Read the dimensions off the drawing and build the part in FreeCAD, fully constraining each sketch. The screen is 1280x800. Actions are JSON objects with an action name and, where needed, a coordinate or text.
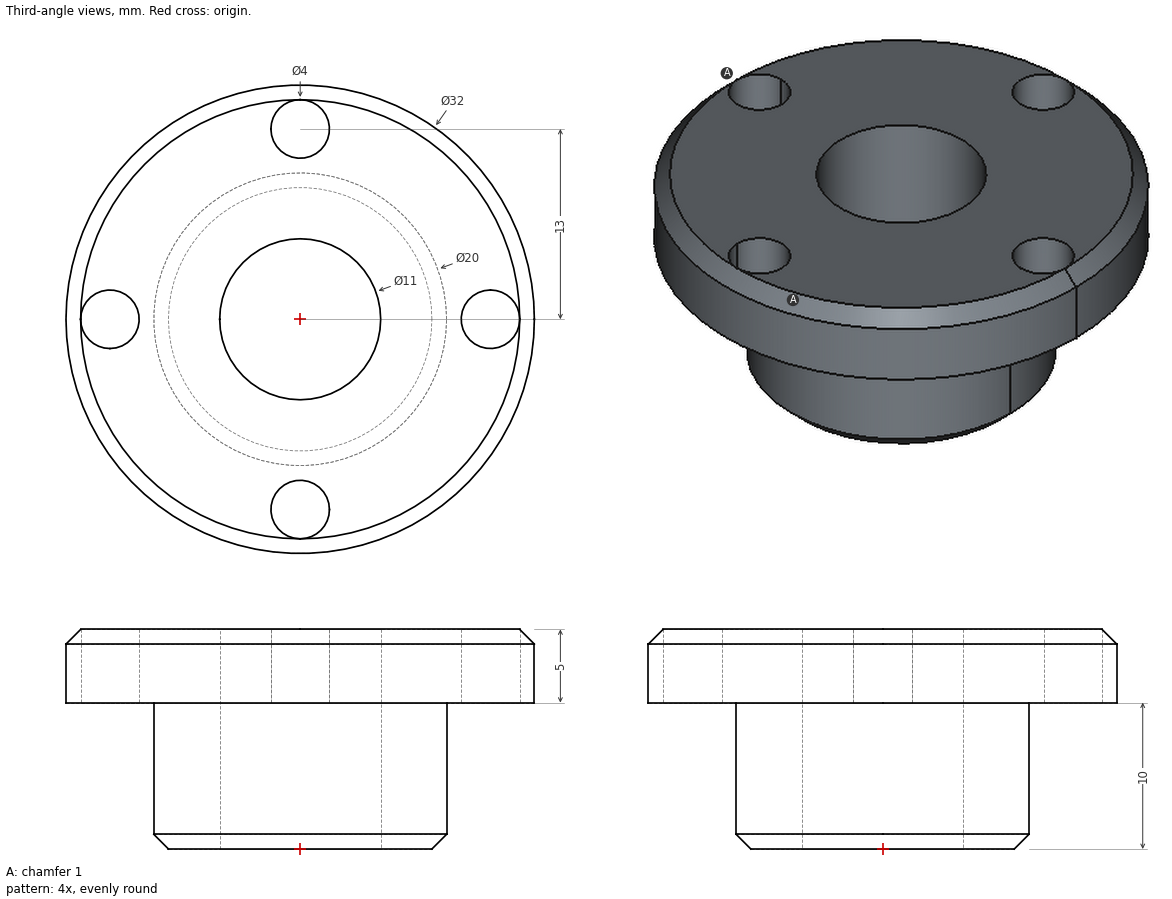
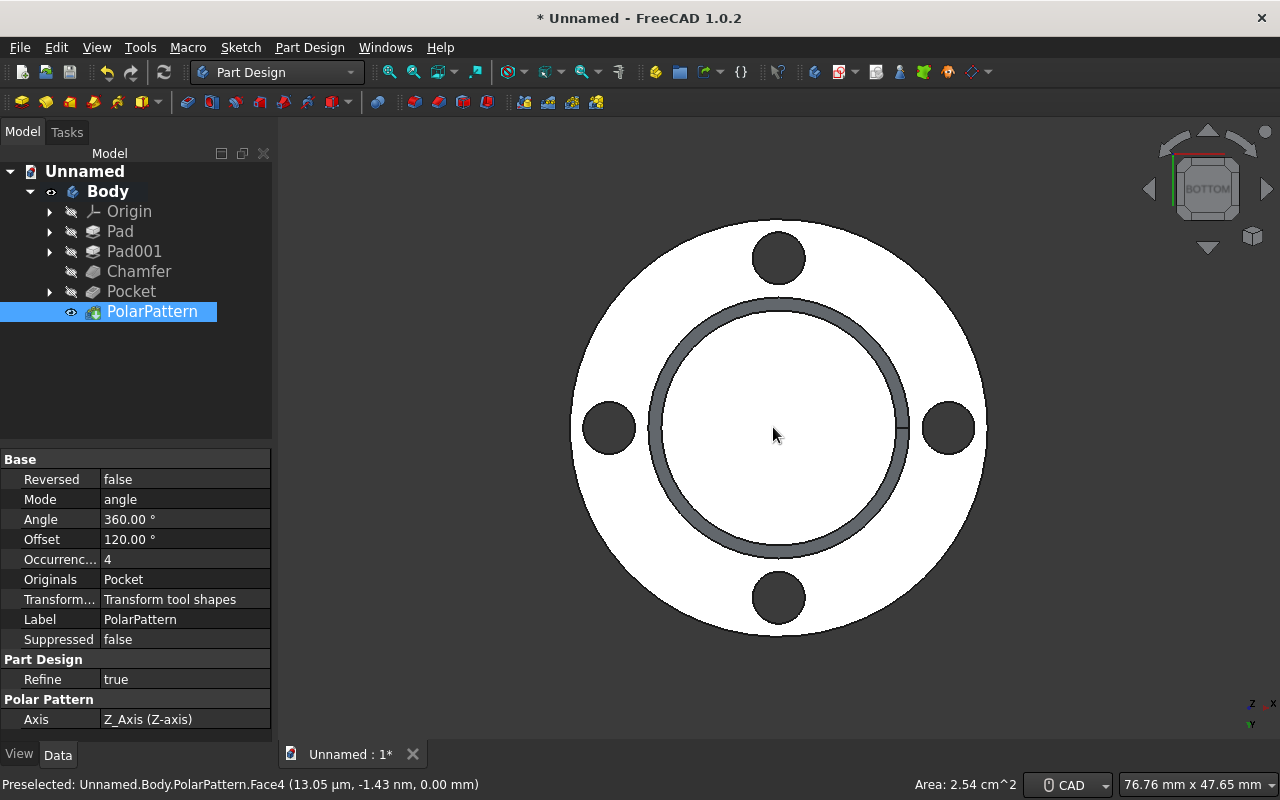
{"action": "left_click", "coordinate": [840, 72]}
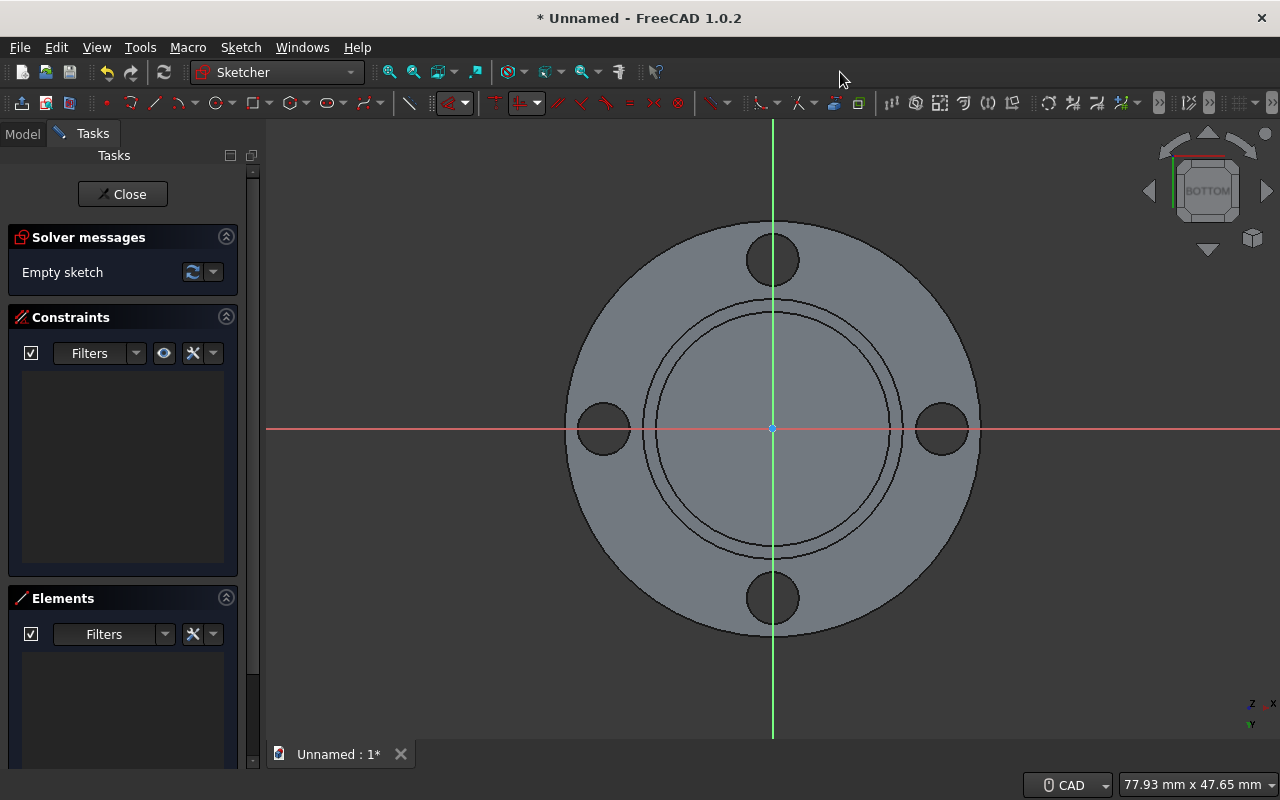
{"action": "scroll", "coordinate": [813, 429], "scroll_direction": "up", "scroll_amount": 5}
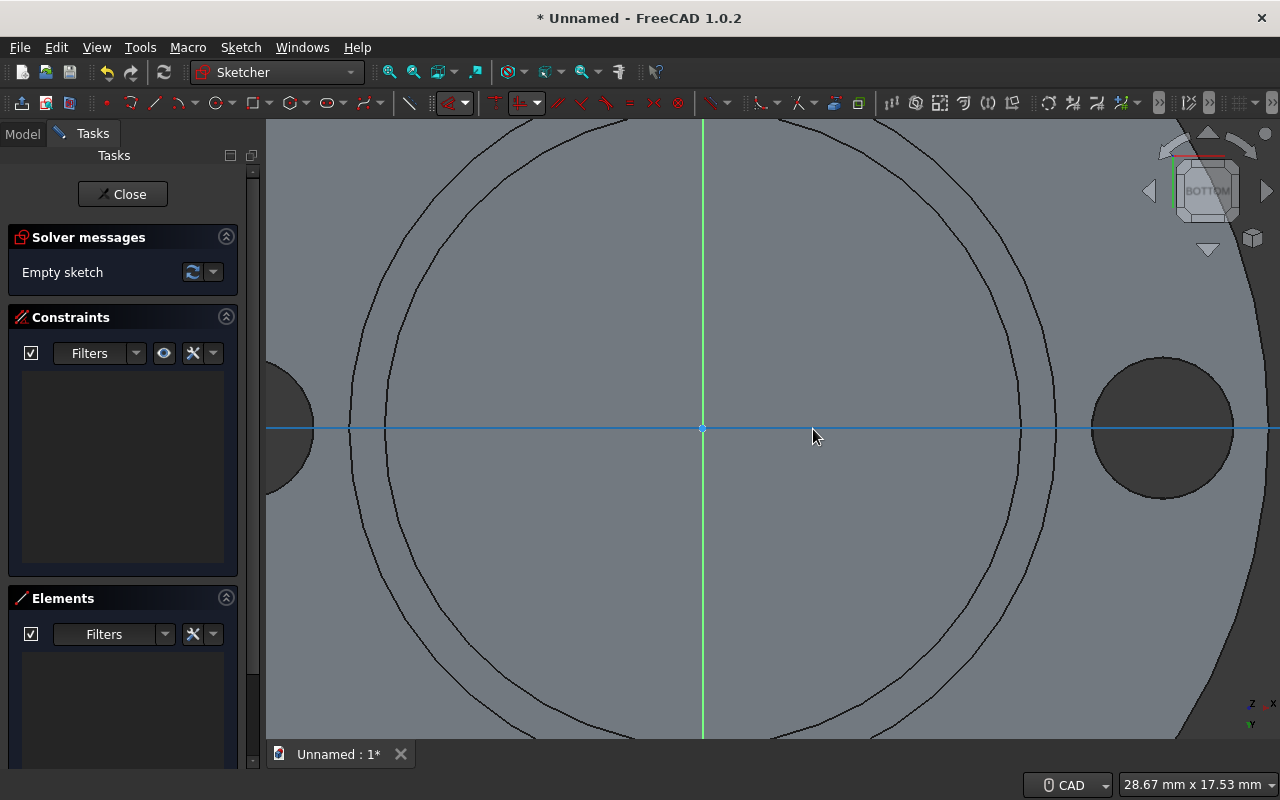
{"action": "left_click", "coordinate": [216, 104]}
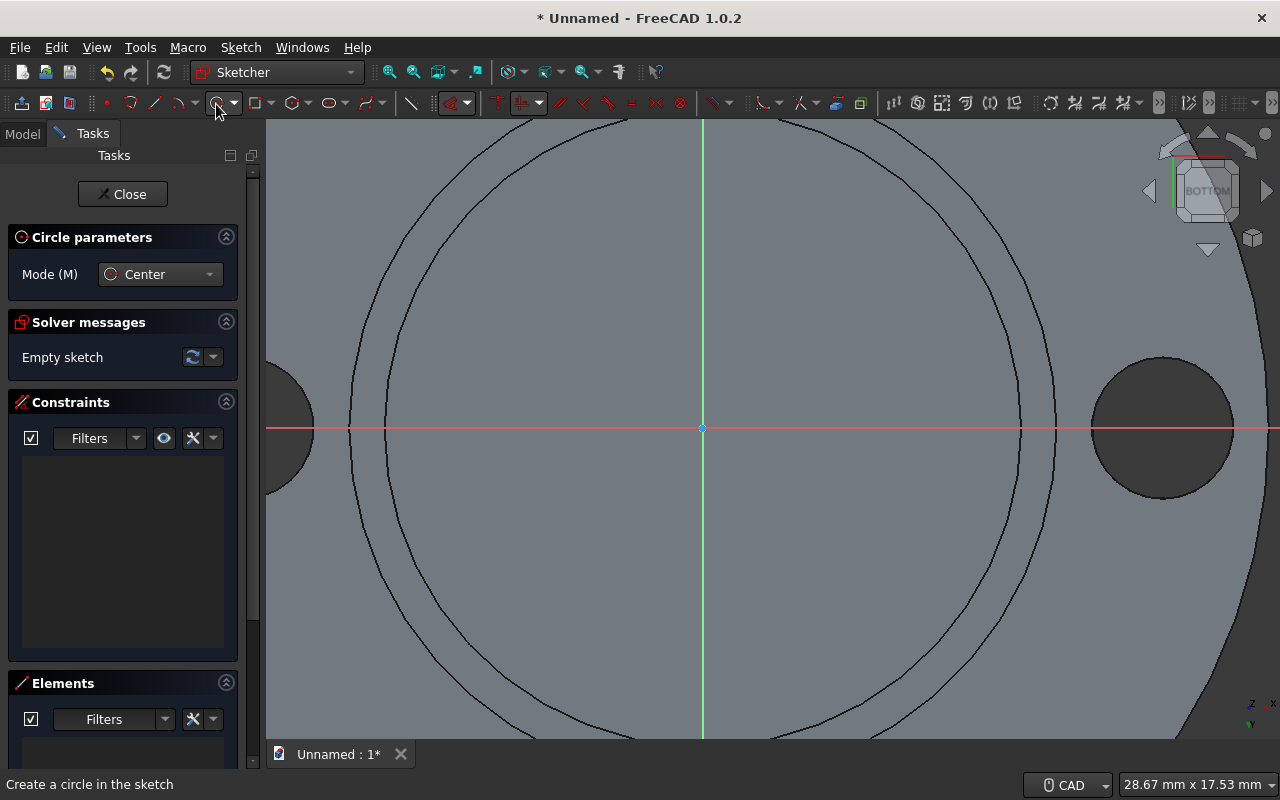
{"action": "left_click", "coordinate": [703, 428]}
{"action": "left_click", "coordinate": [840, 291]}
{"action": "key", "text": "Escape"}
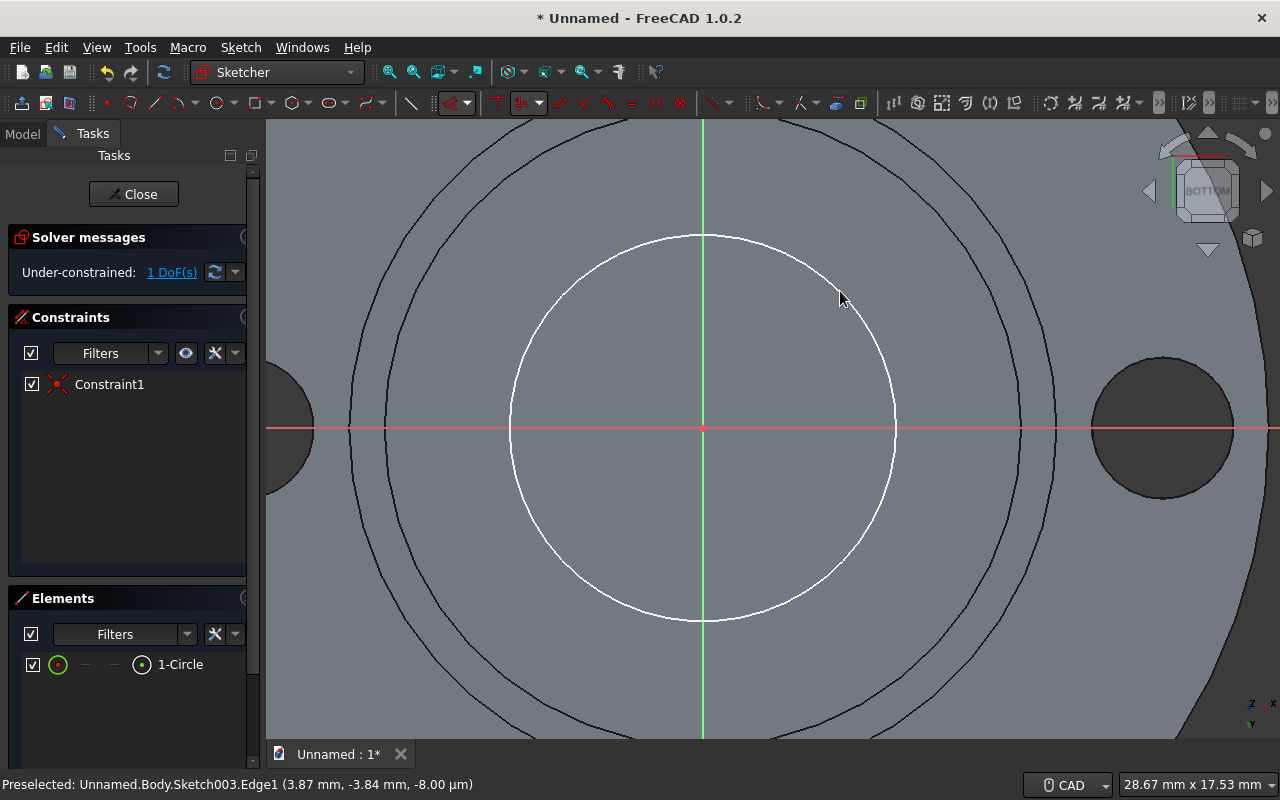
{"action": "left_click", "coordinate": [839, 291]}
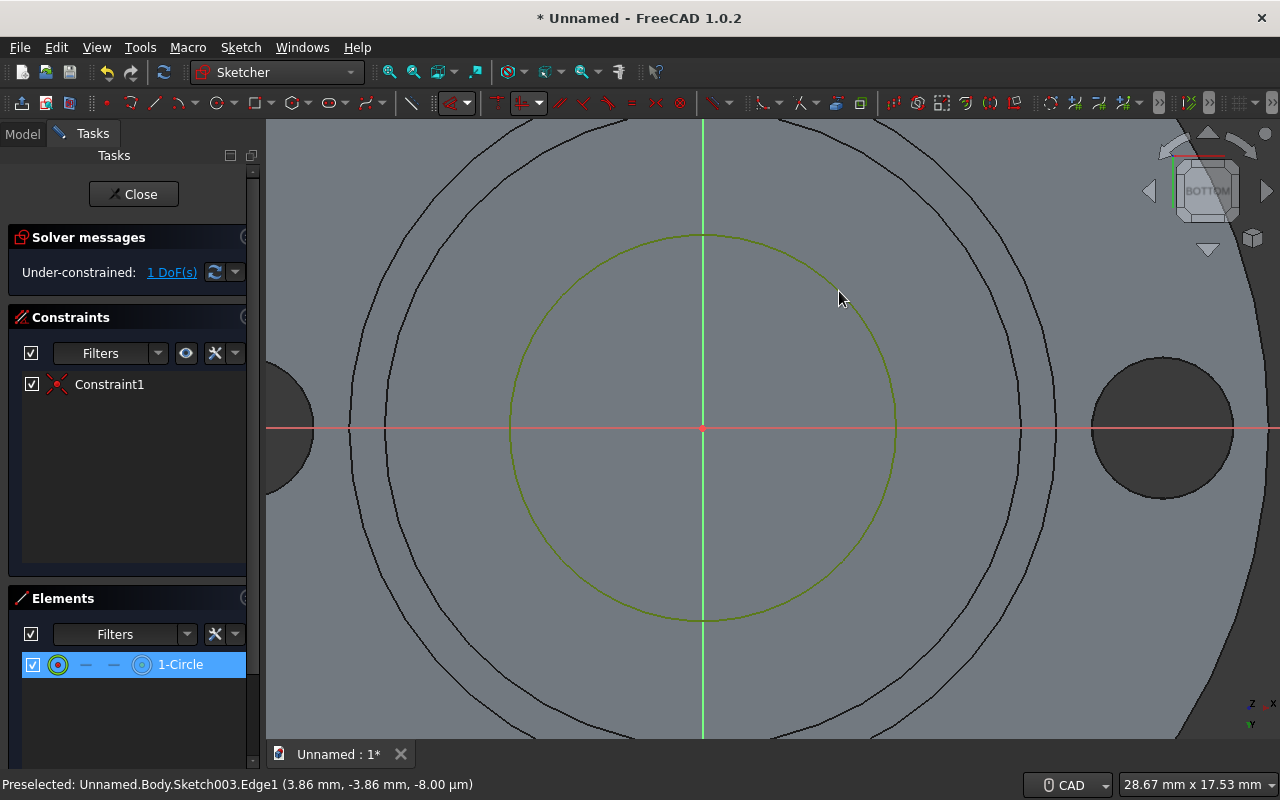
{"action": "left_click", "coordinate": [470, 104]}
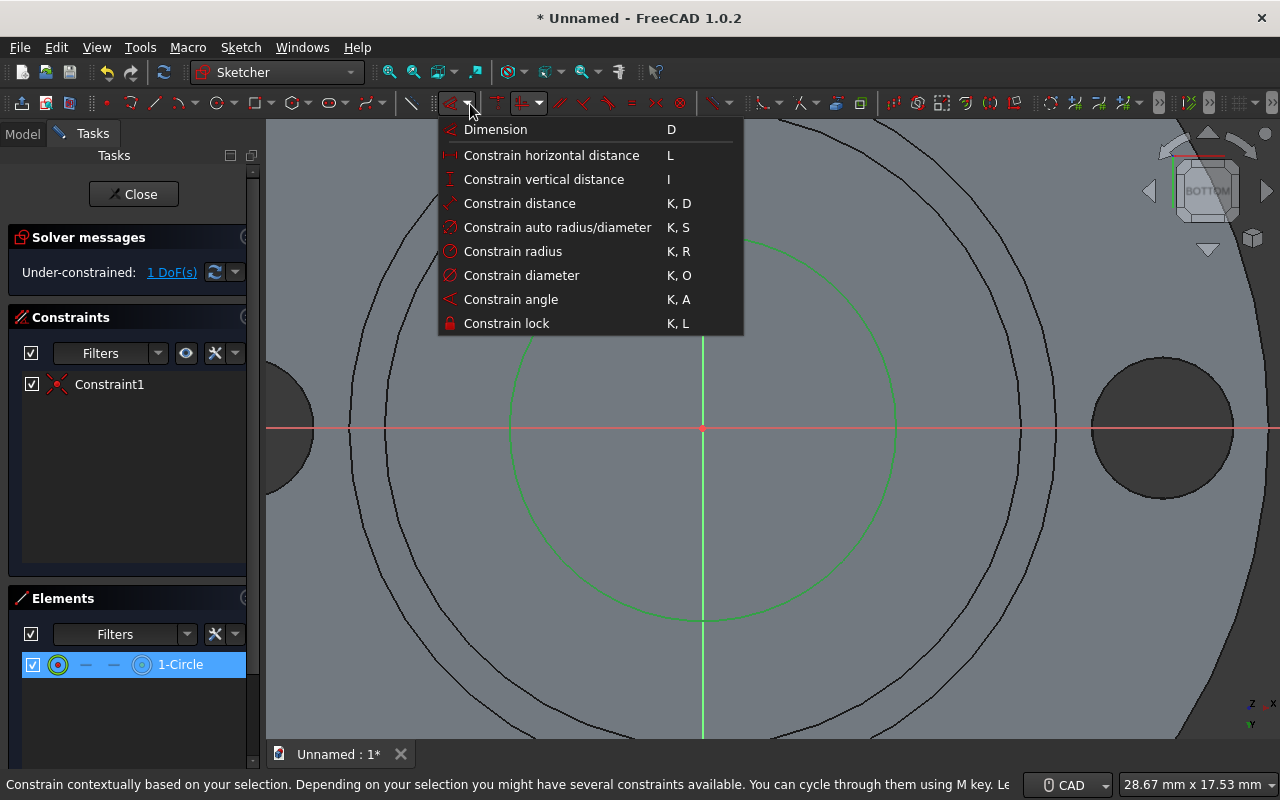
{"action": "left_click", "coordinate": [591, 275]}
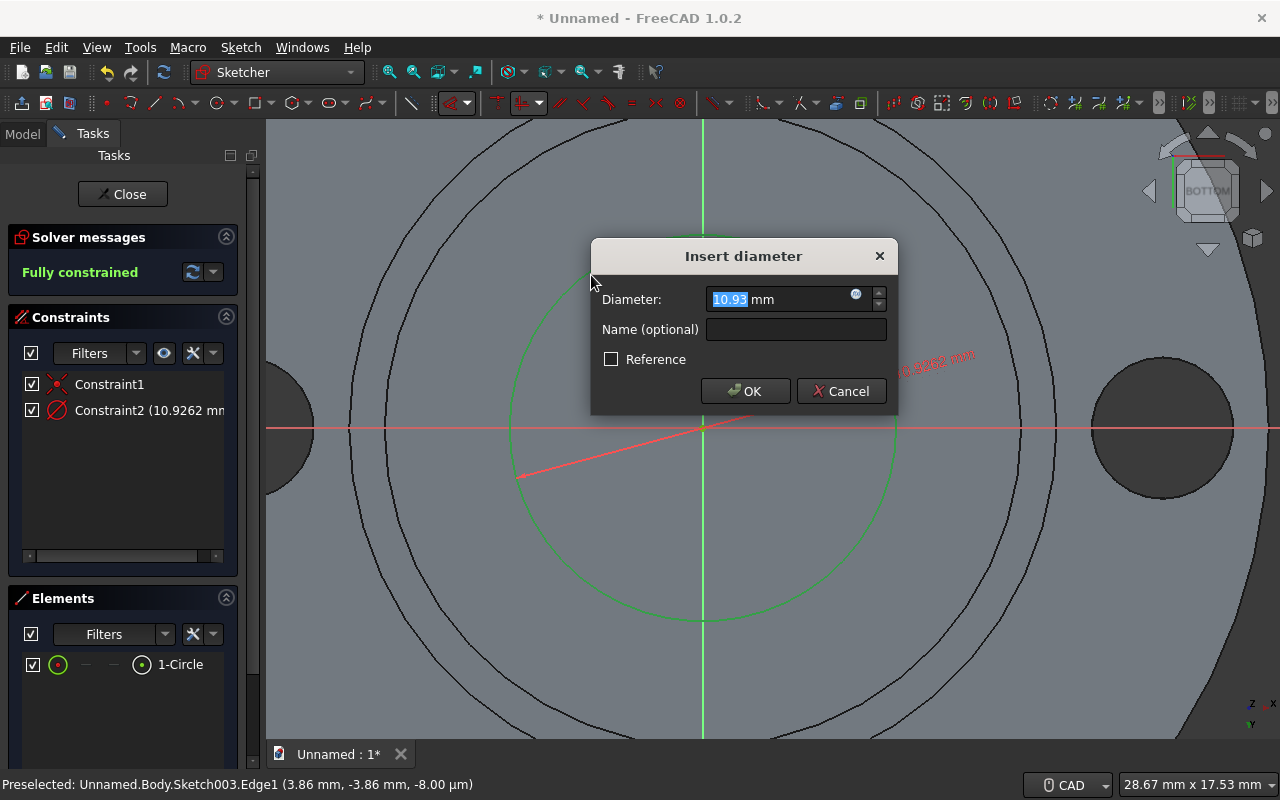
{"action": "type", "text": "11"}
{"action": "key", "text": "Return"}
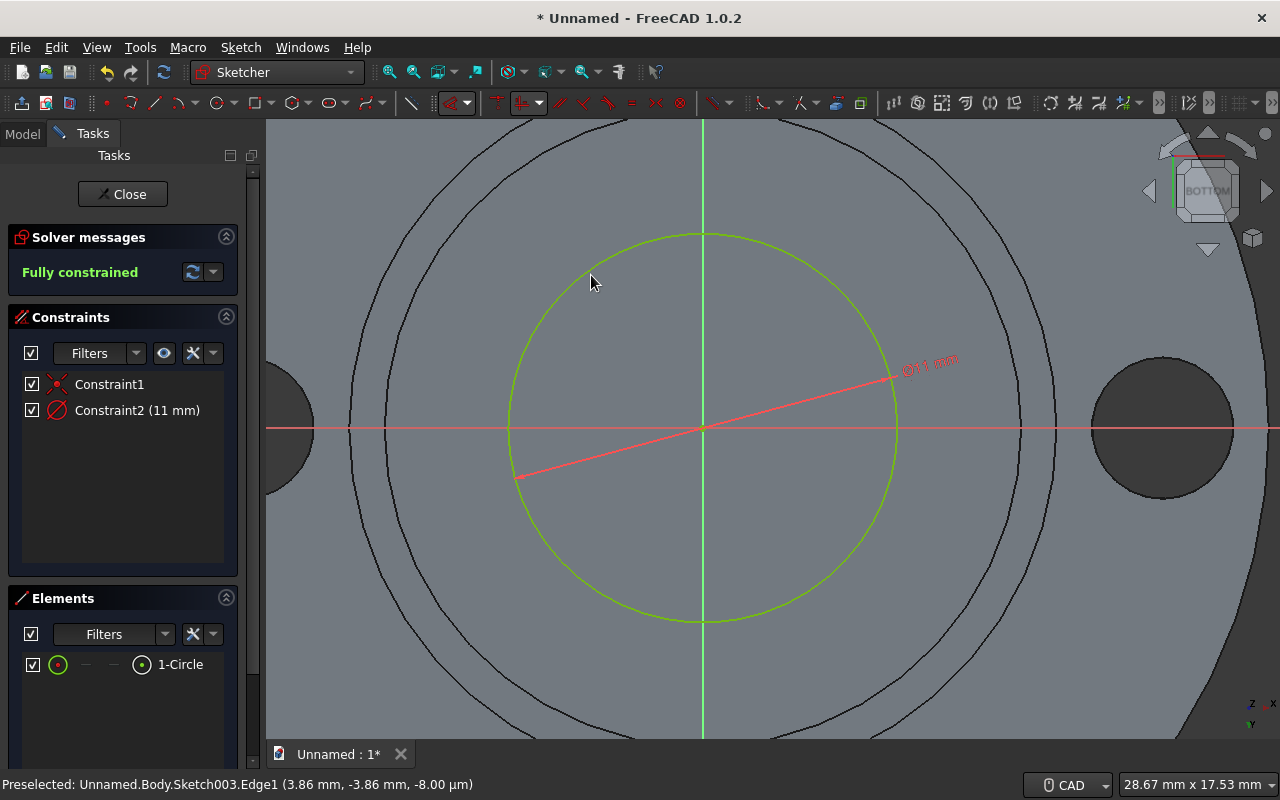
{"action": "left_click", "coordinate": [123, 194]}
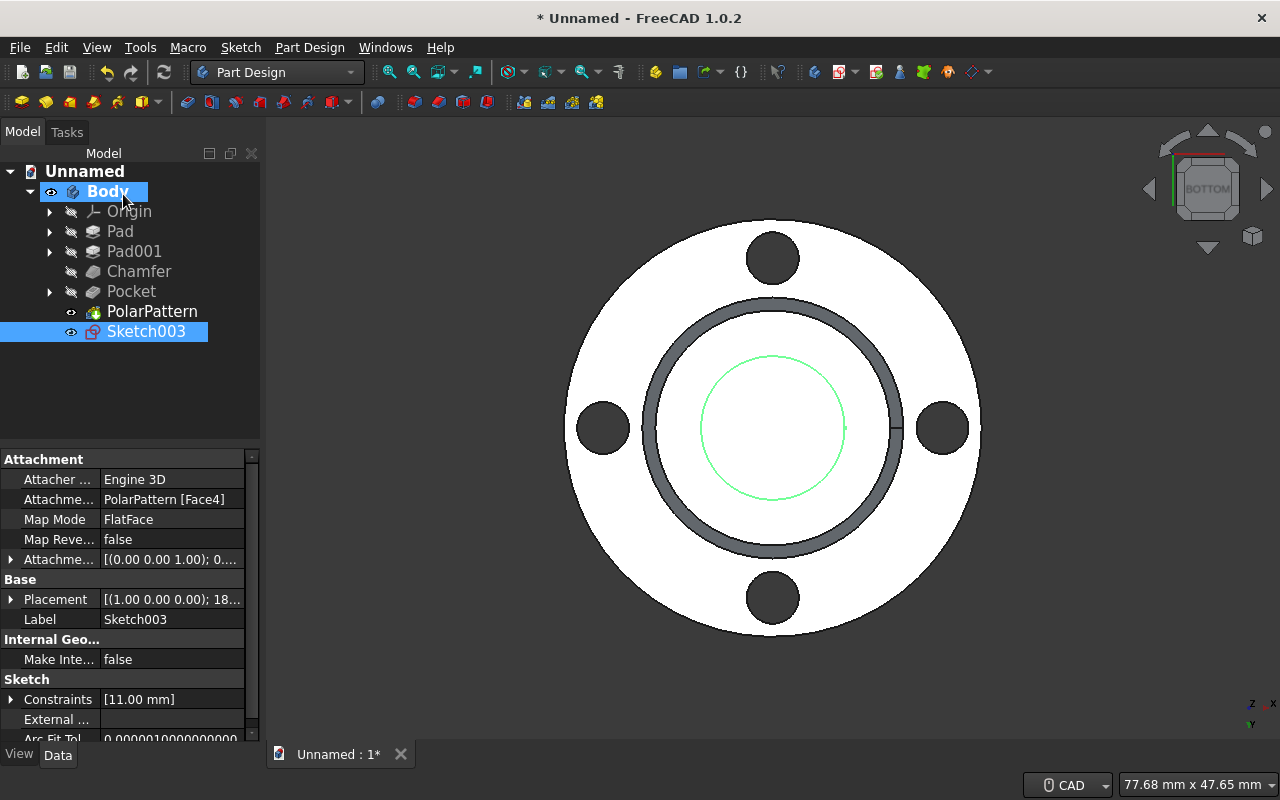
{"action": "left_click", "coordinate": [188, 102]}